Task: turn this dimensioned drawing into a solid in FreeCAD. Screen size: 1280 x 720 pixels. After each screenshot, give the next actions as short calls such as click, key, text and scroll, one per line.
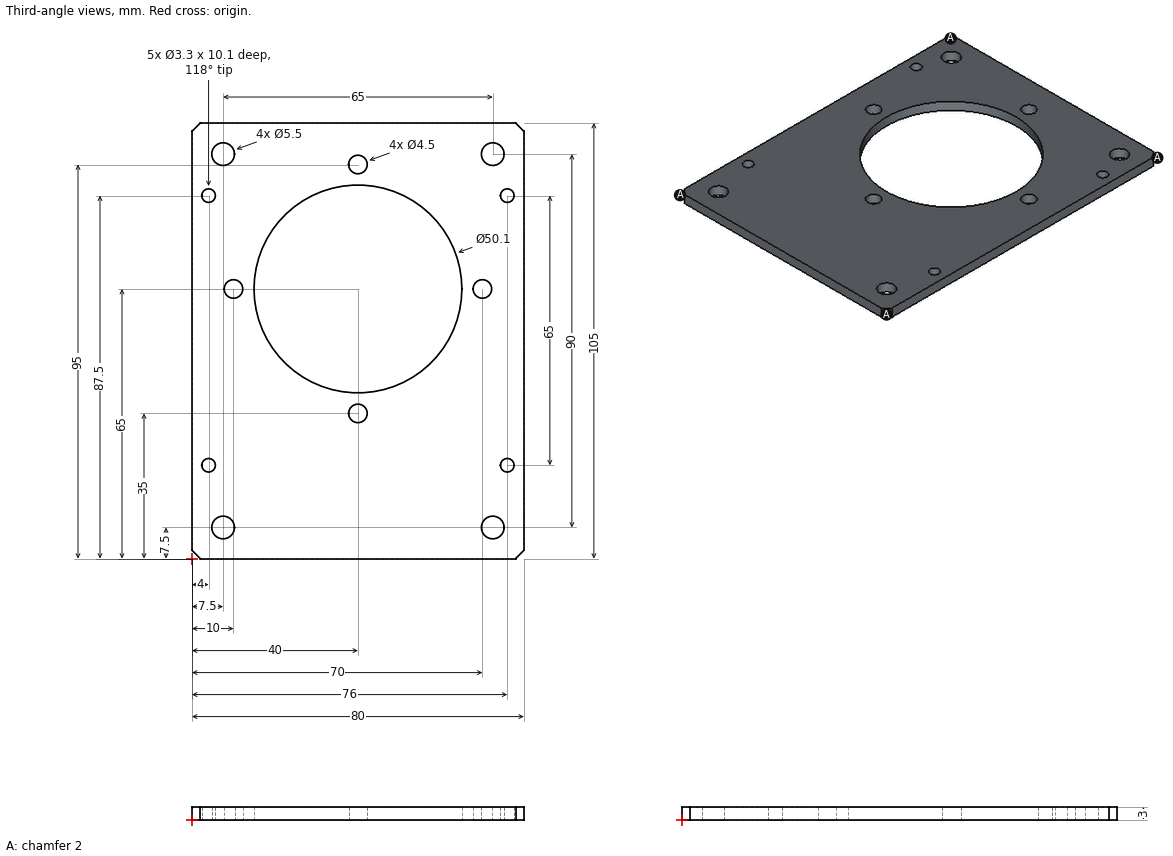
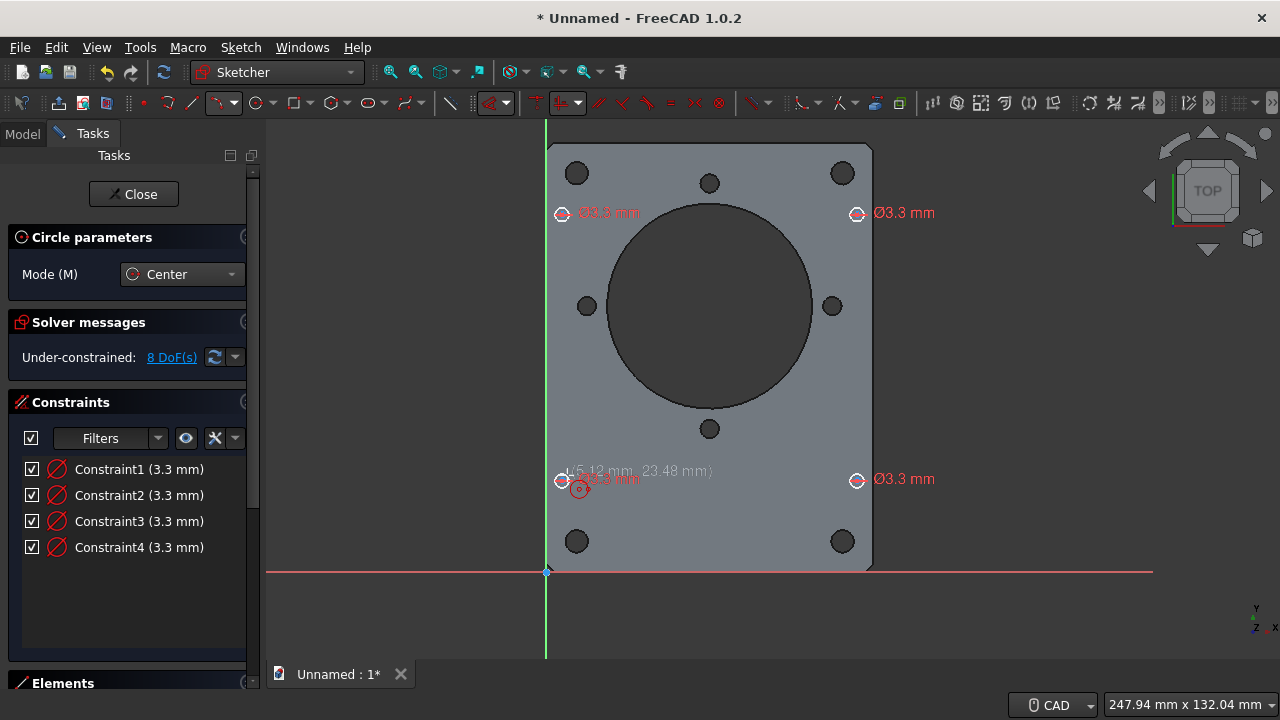
scroll(710, 306, up, 7)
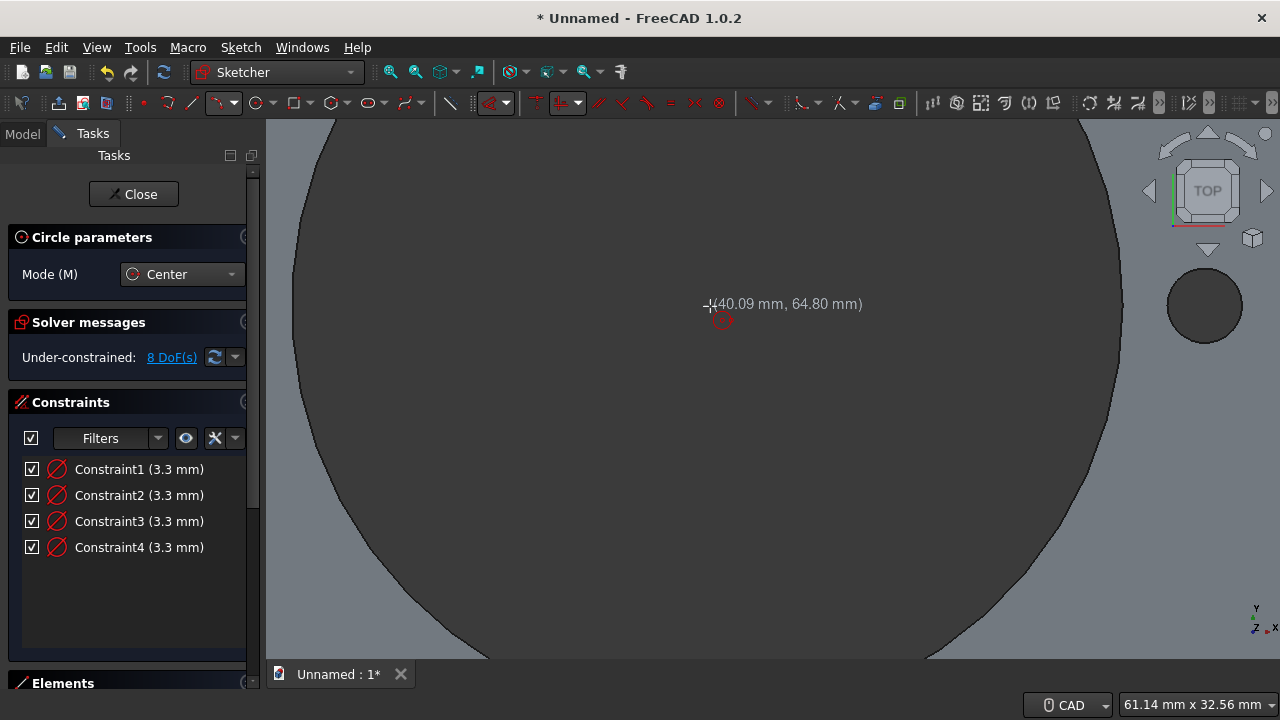
scroll(710, 305, down, 7)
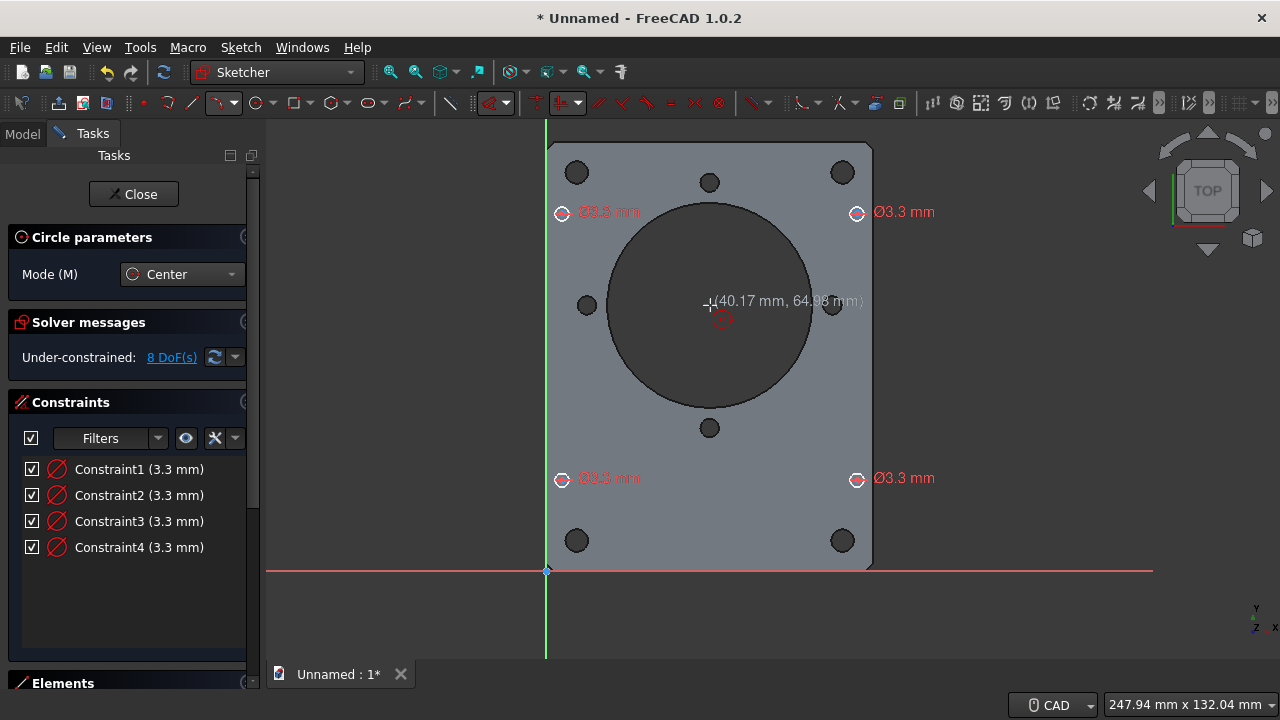
click(710, 305)
move(714, 301)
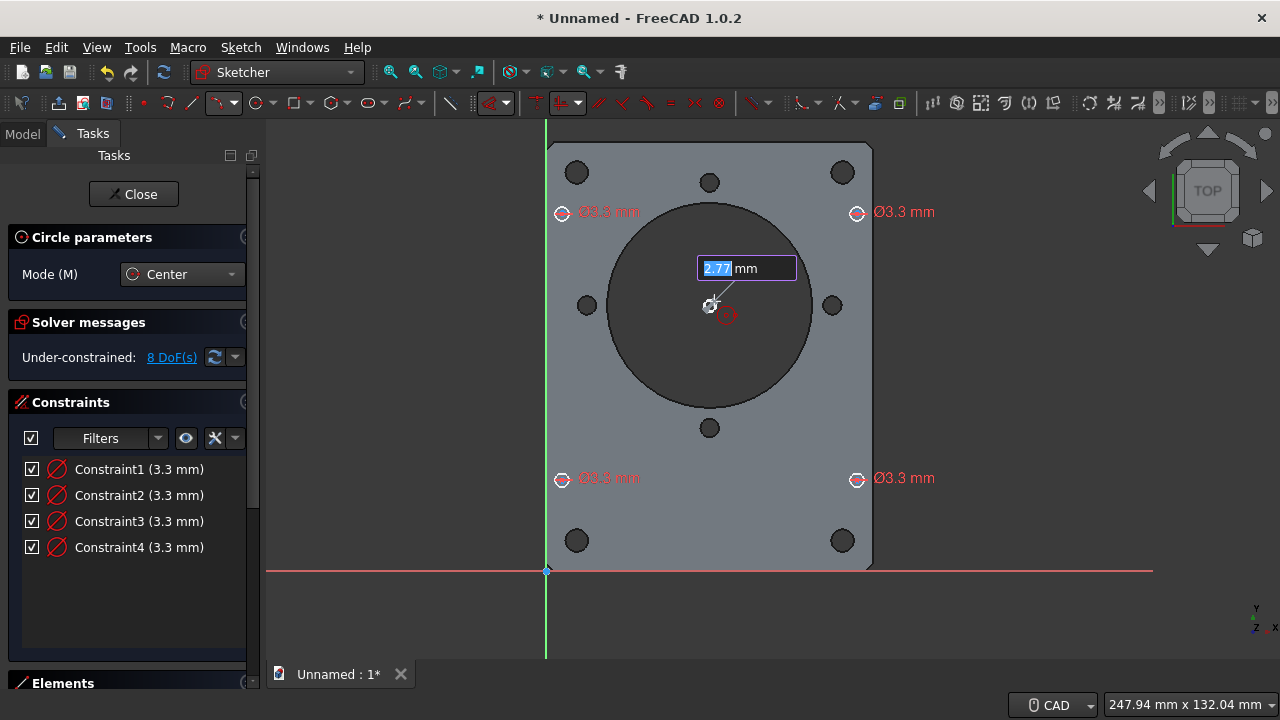
text(3.3)
key(Return)
key(Escape)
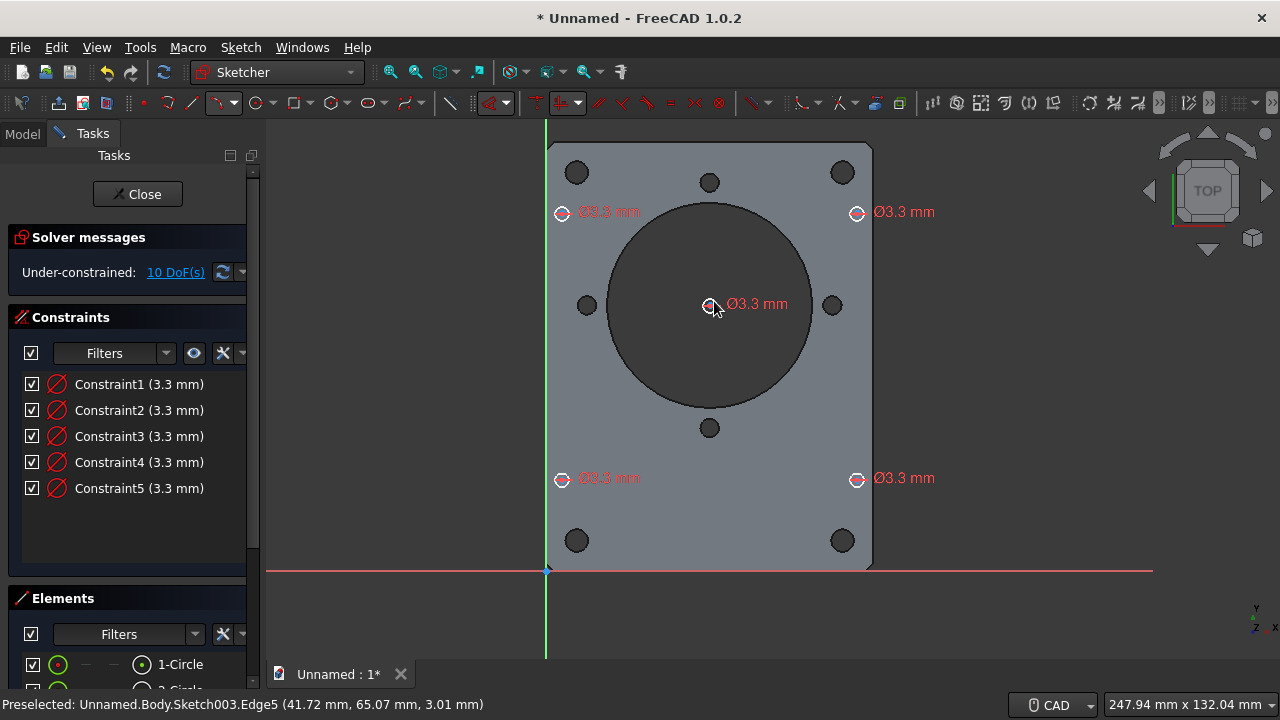
click(562, 214)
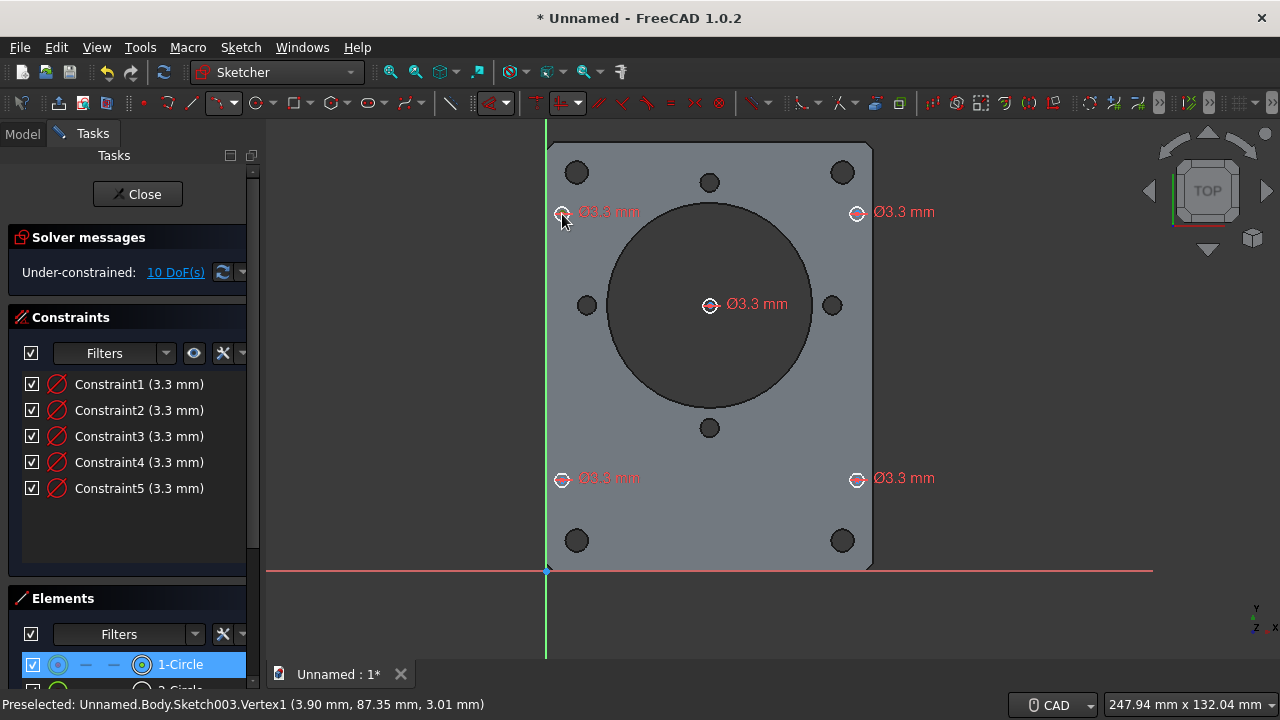
click(857, 214)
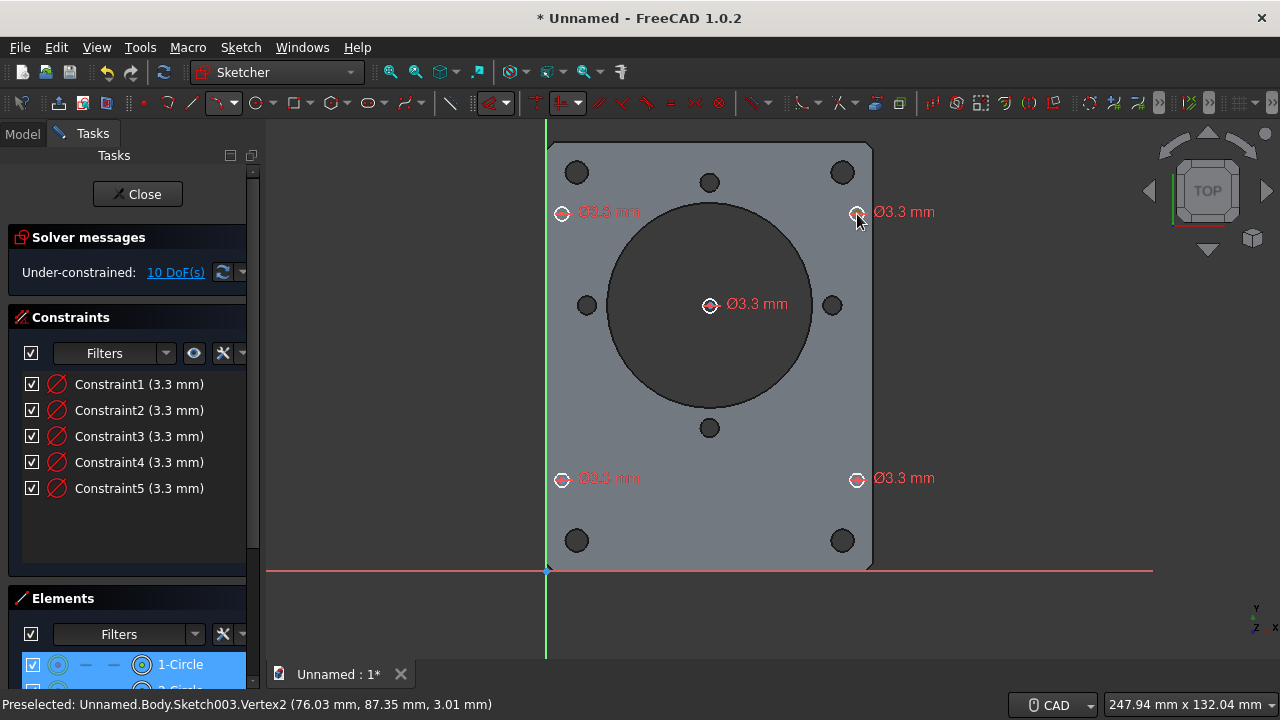
key(h)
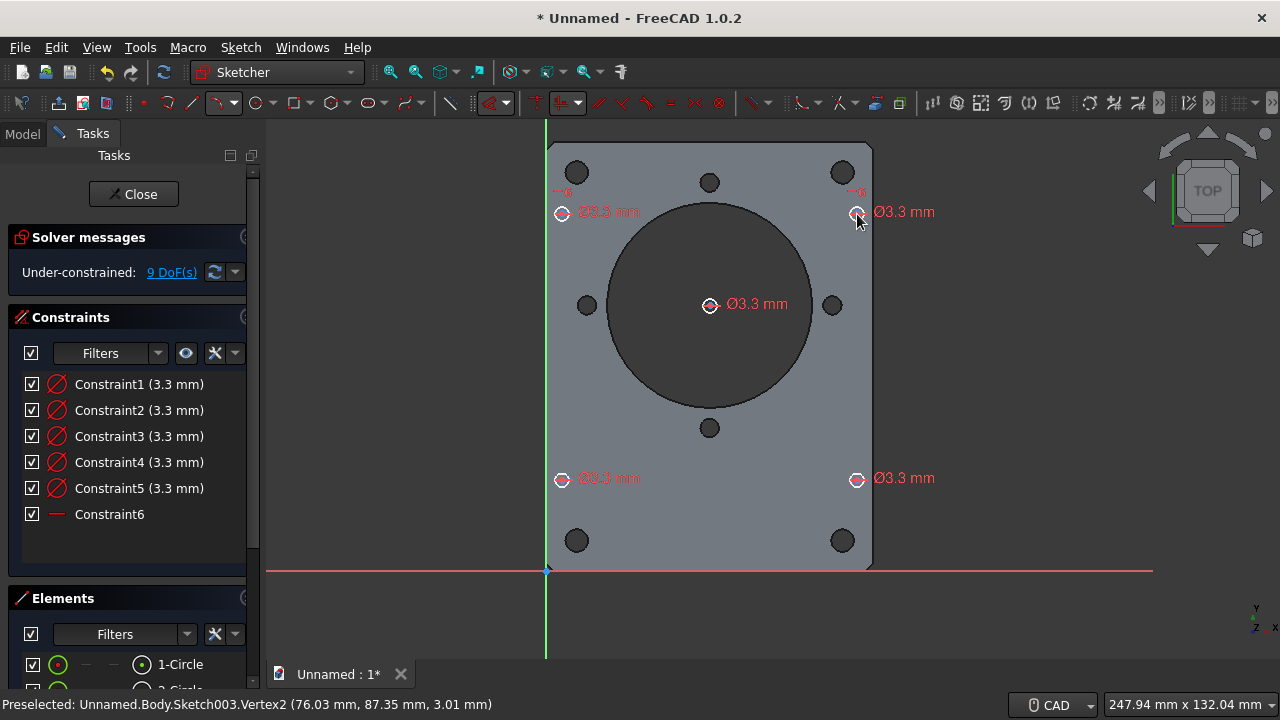
click(857, 214)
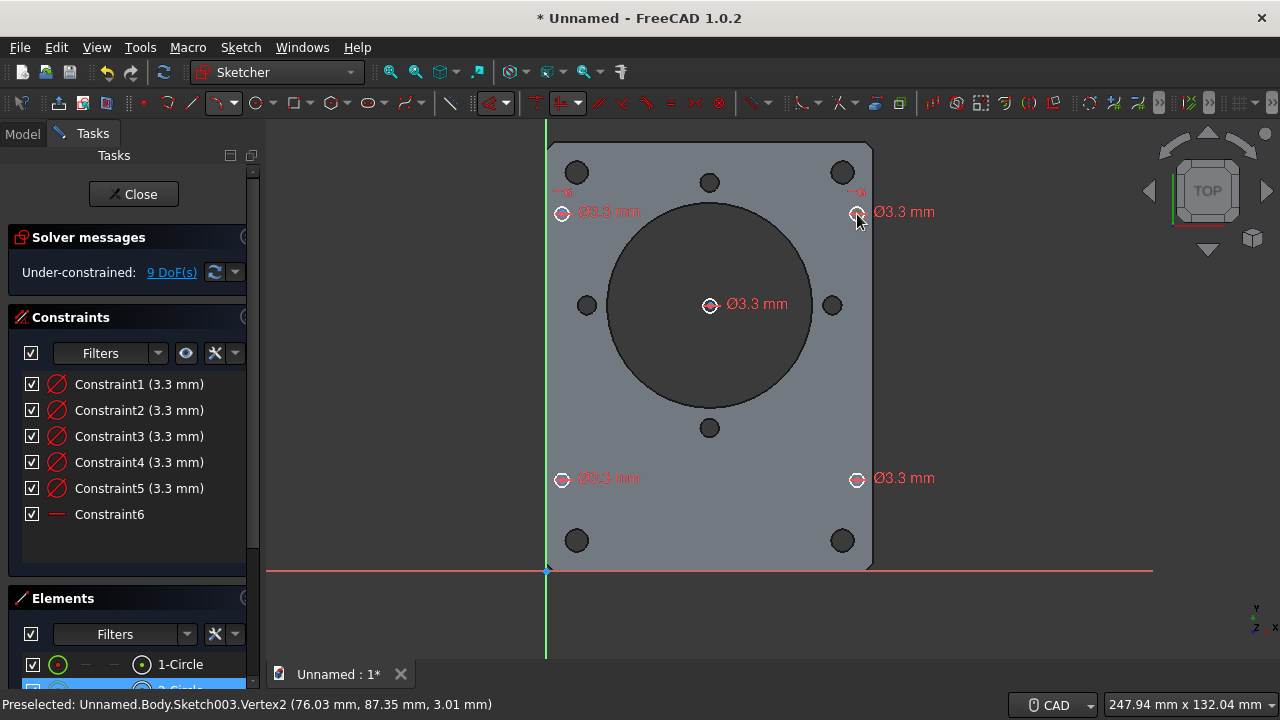
click(857, 480)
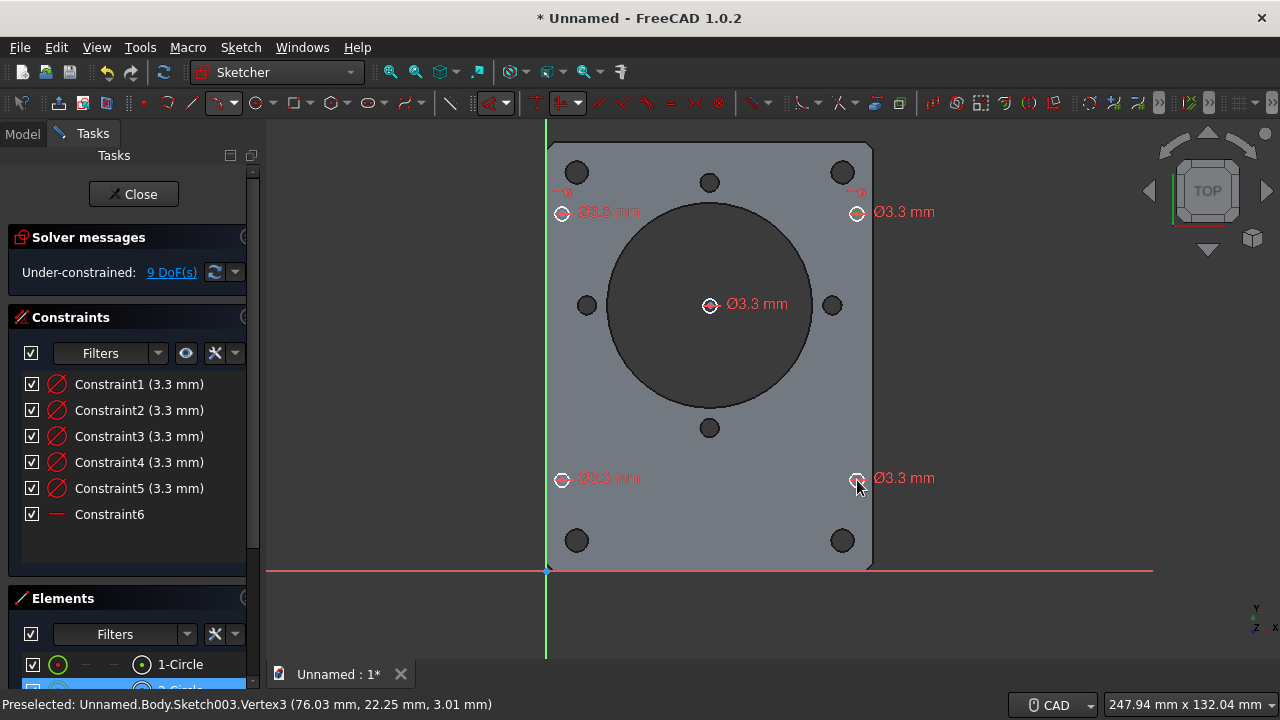
click(580, 104)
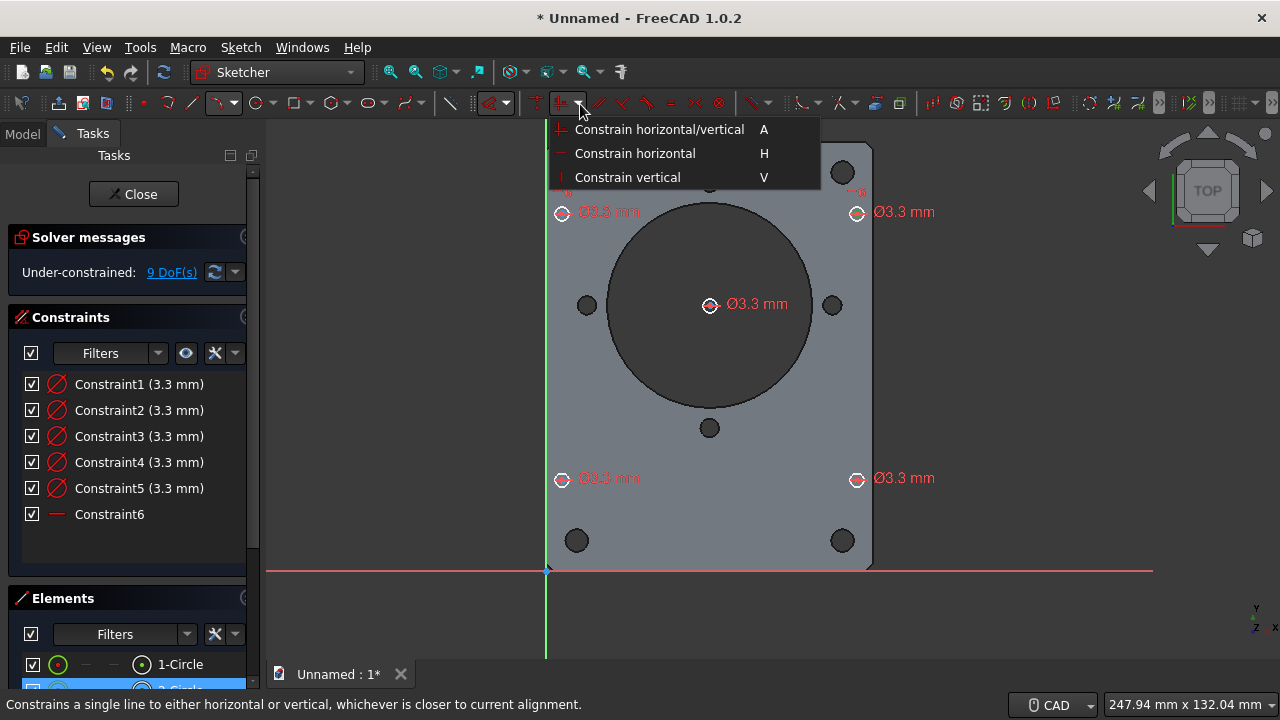
click(685, 177)